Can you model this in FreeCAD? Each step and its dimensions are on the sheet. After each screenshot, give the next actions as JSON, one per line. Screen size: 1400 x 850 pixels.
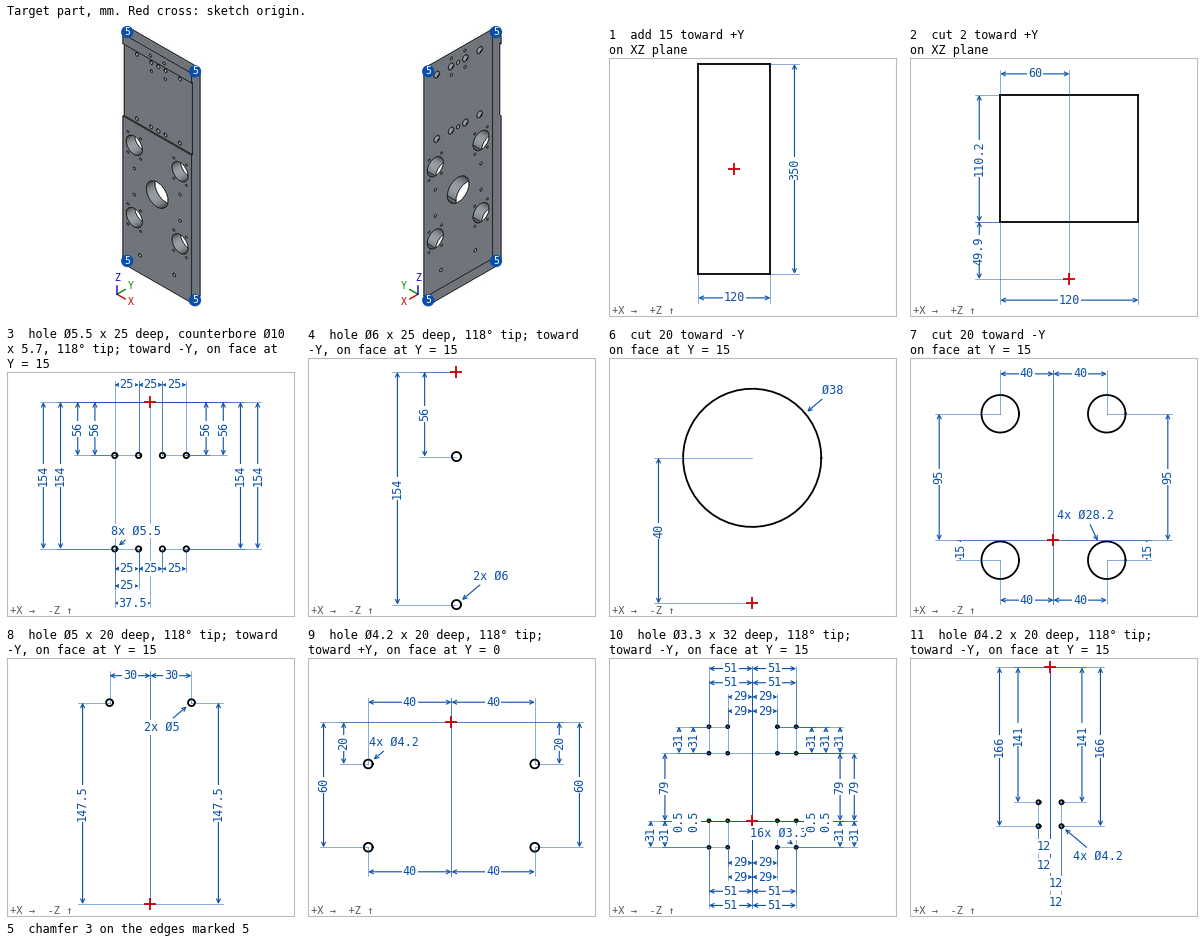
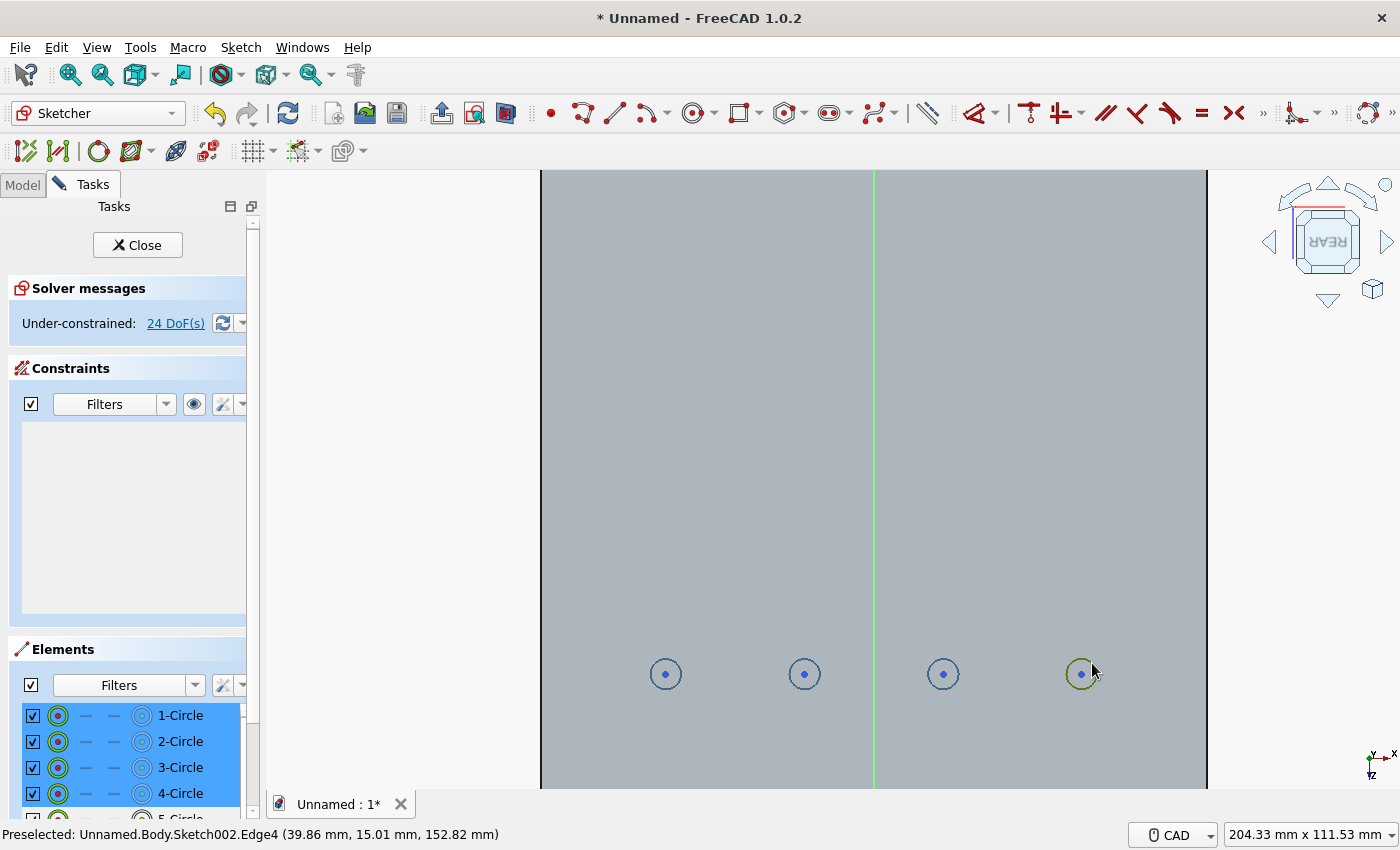
{"action": "scroll", "coordinate": [675, 664], "scroll_direction": "down", "scroll_amount": 4}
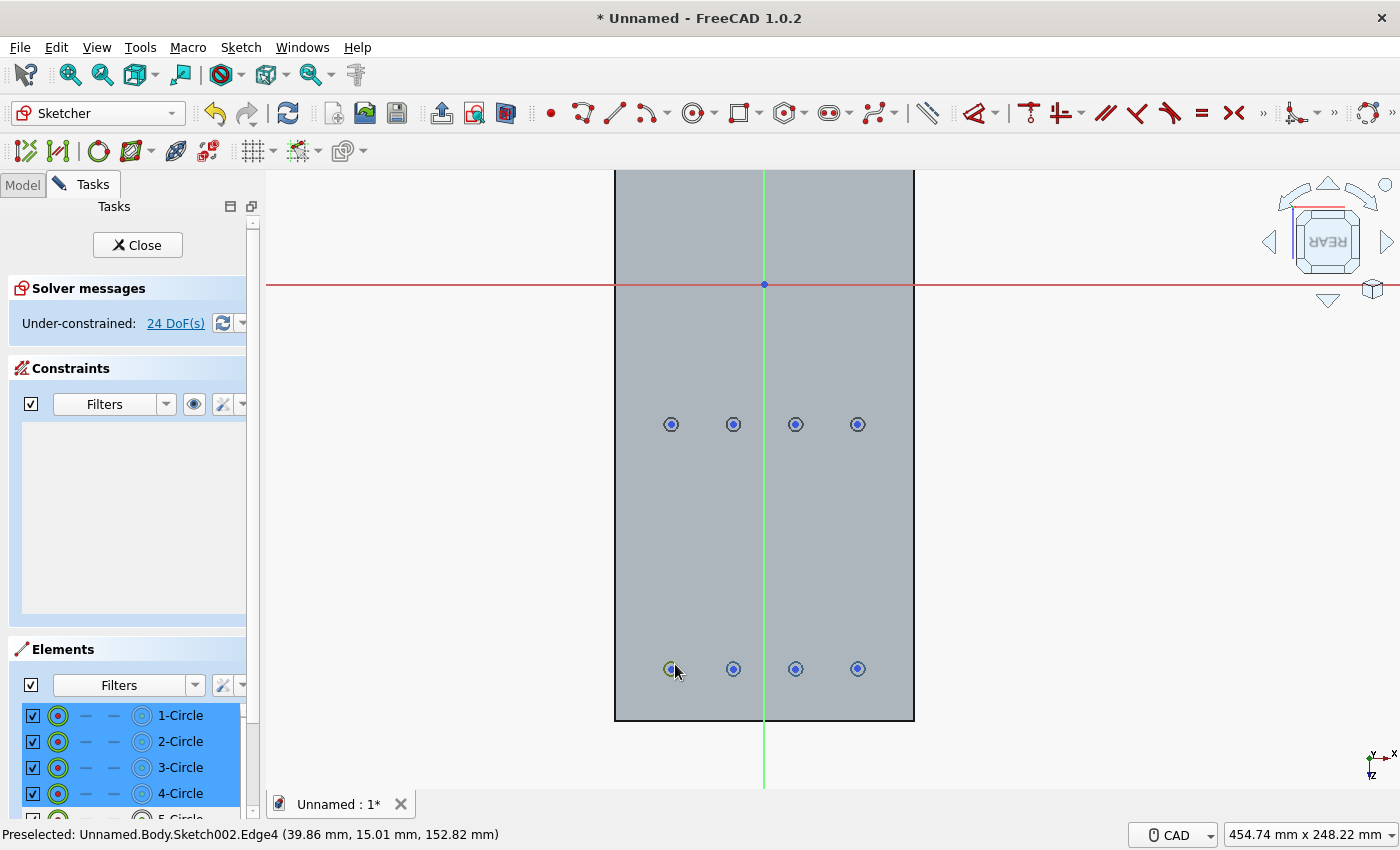
{"action": "scroll", "coordinate": [676, 420], "scroll_direction": "up", "scroll_amount": 4}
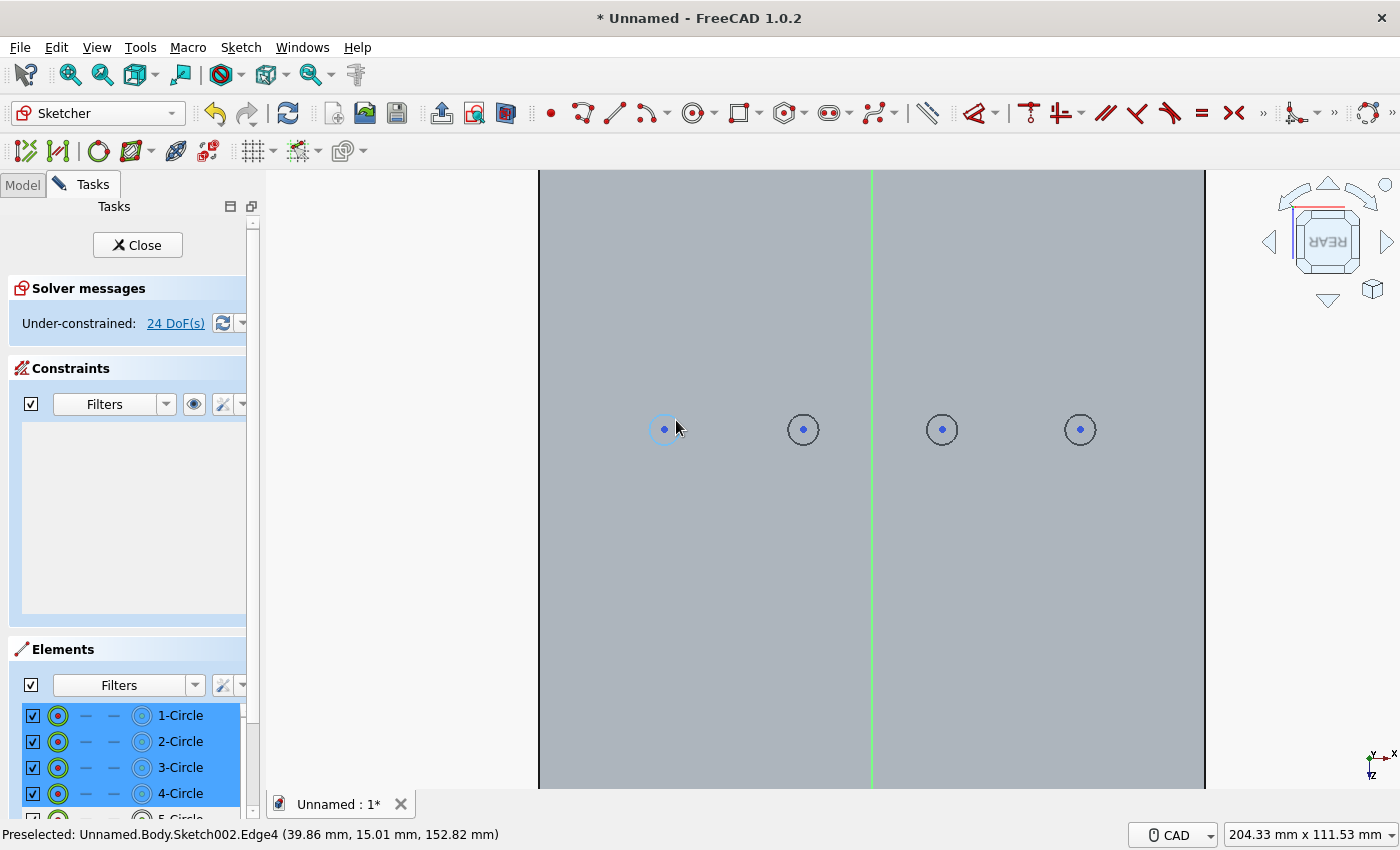
{"action": "left_click", "coordinate": [675, 419]}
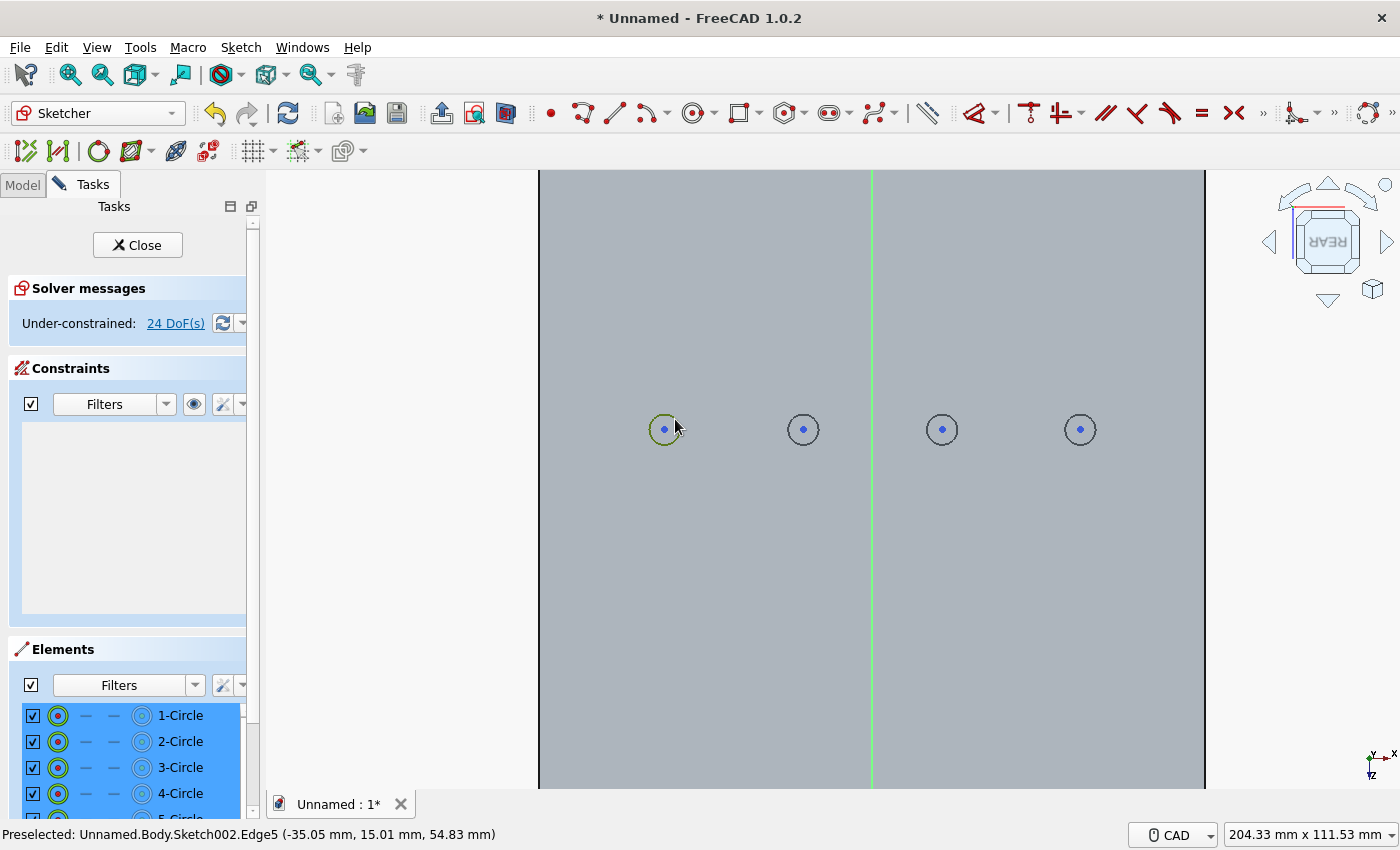
{"action": "left_click", "coordinate": [814, 419]}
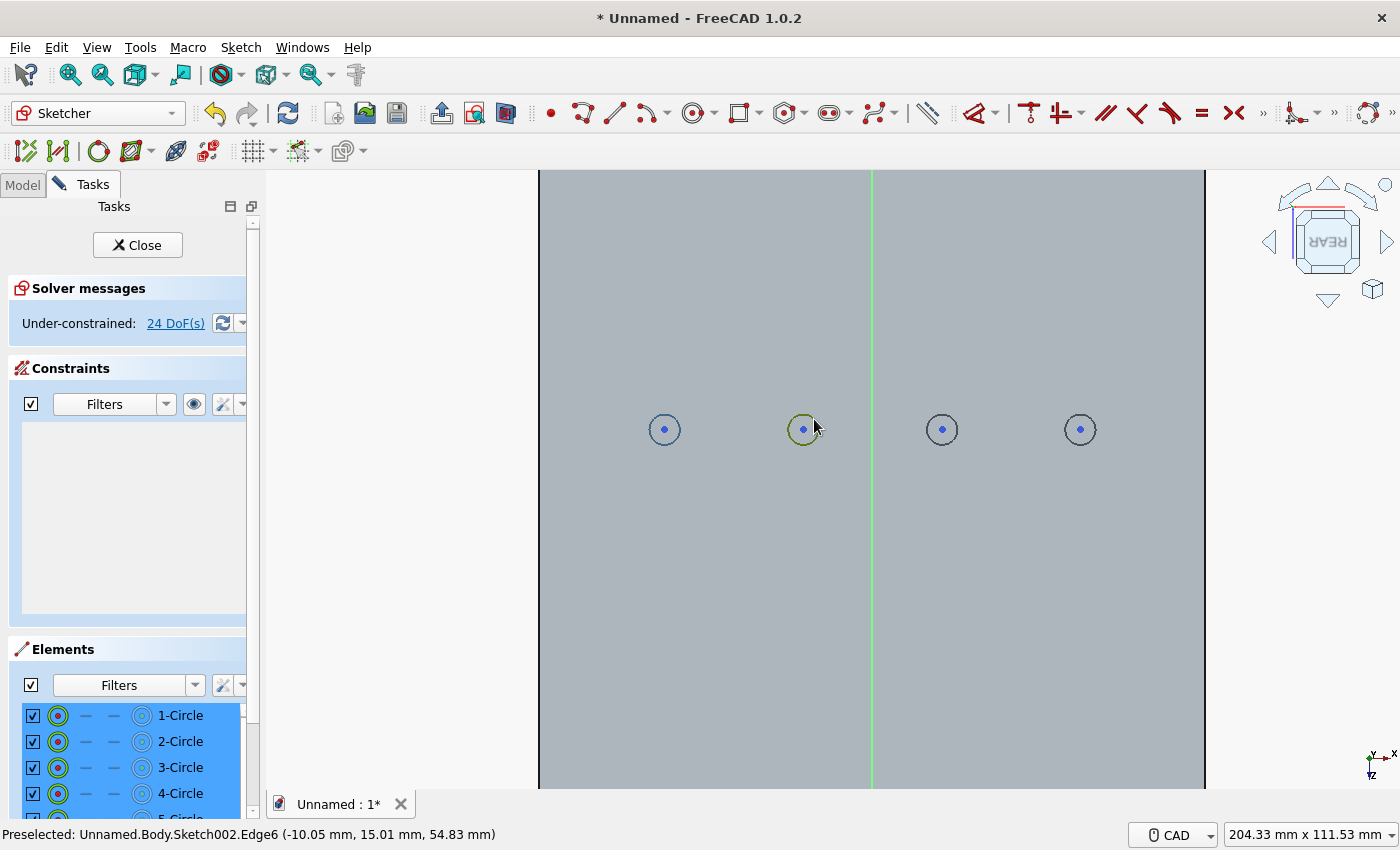
{"action": "left_click", "coordinate": [953, 419]}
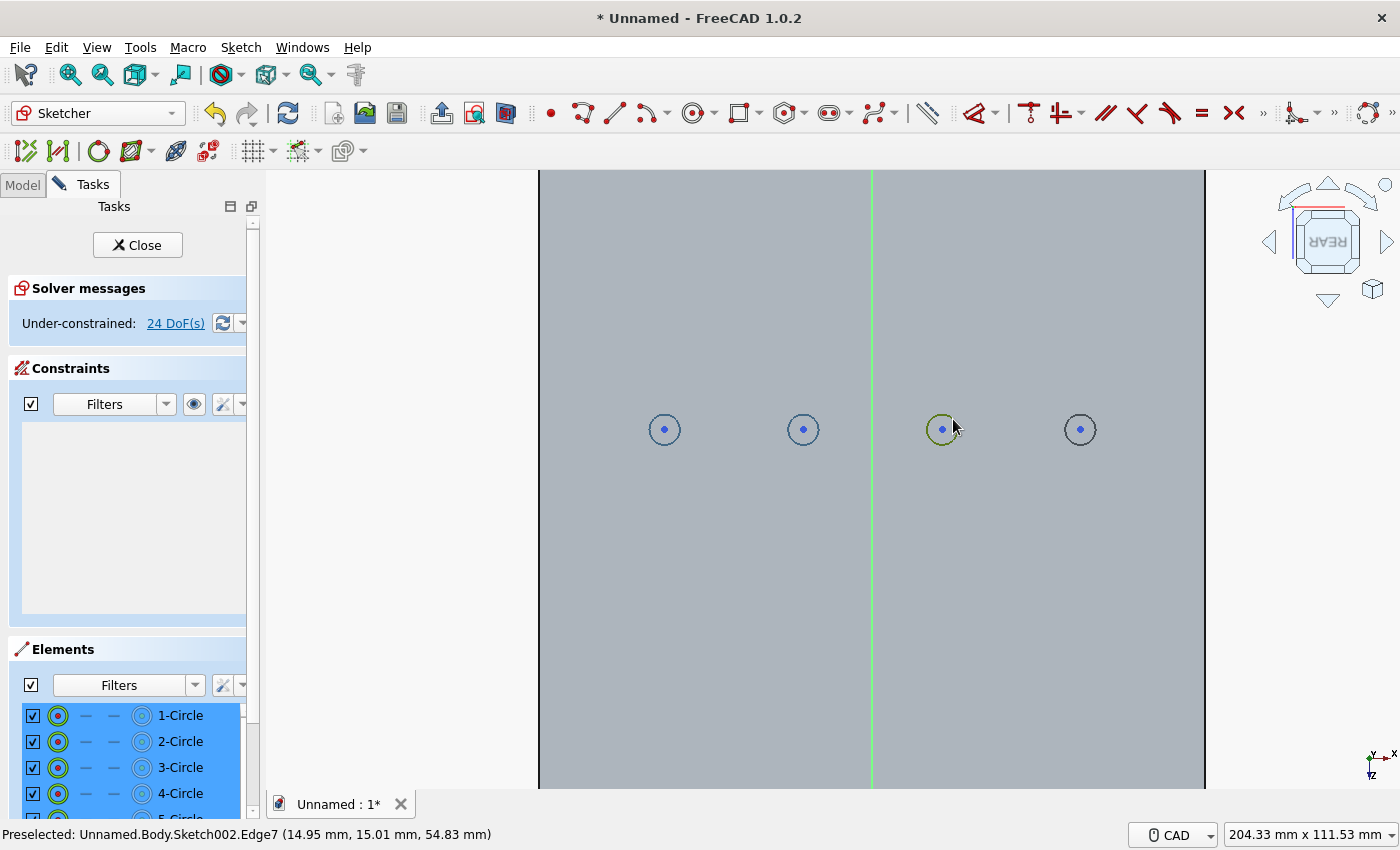
{"action": "left_click", "coordinate": [1091, 419]}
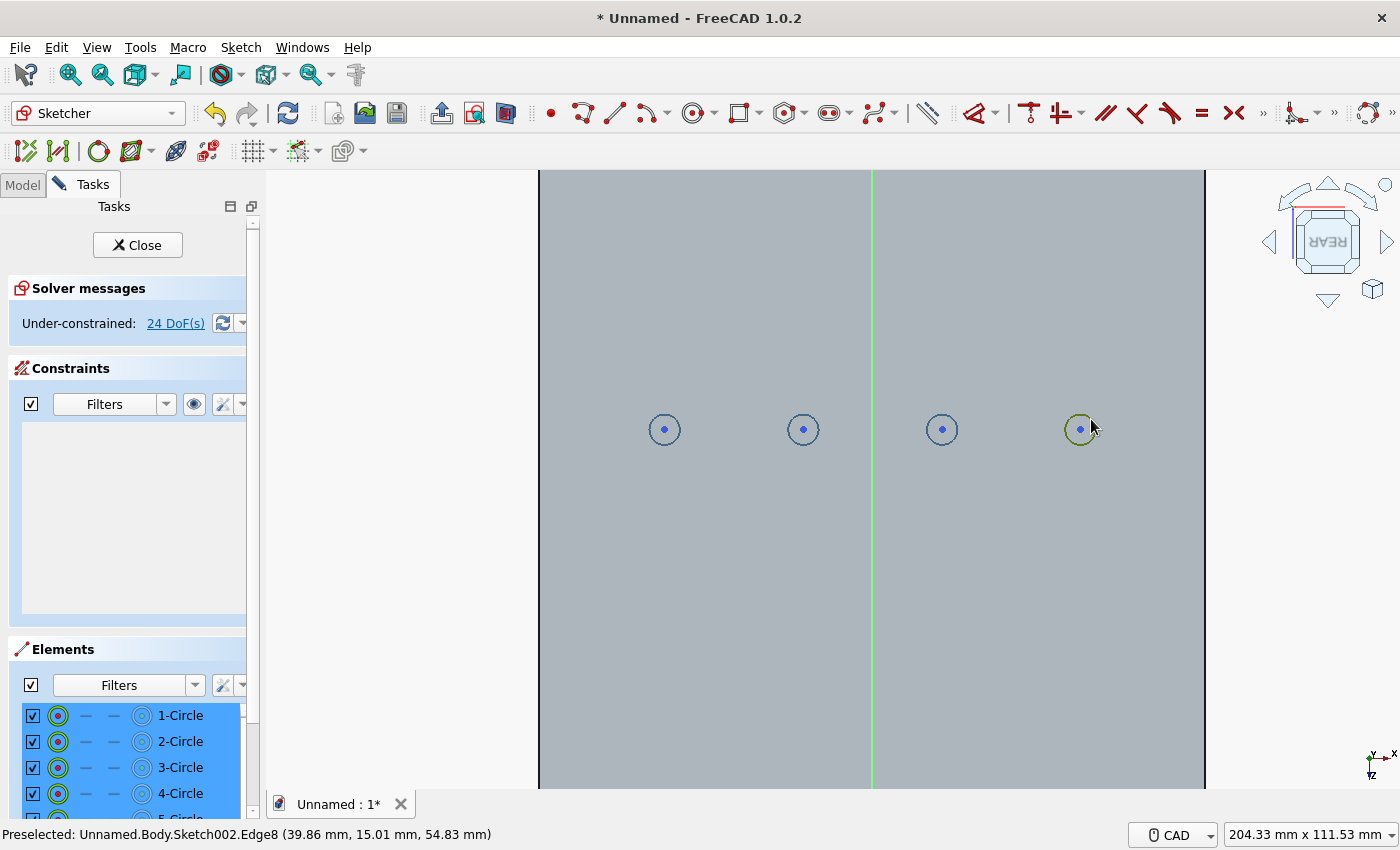
{"action": "left_click", "coordinate": [1202, 114]}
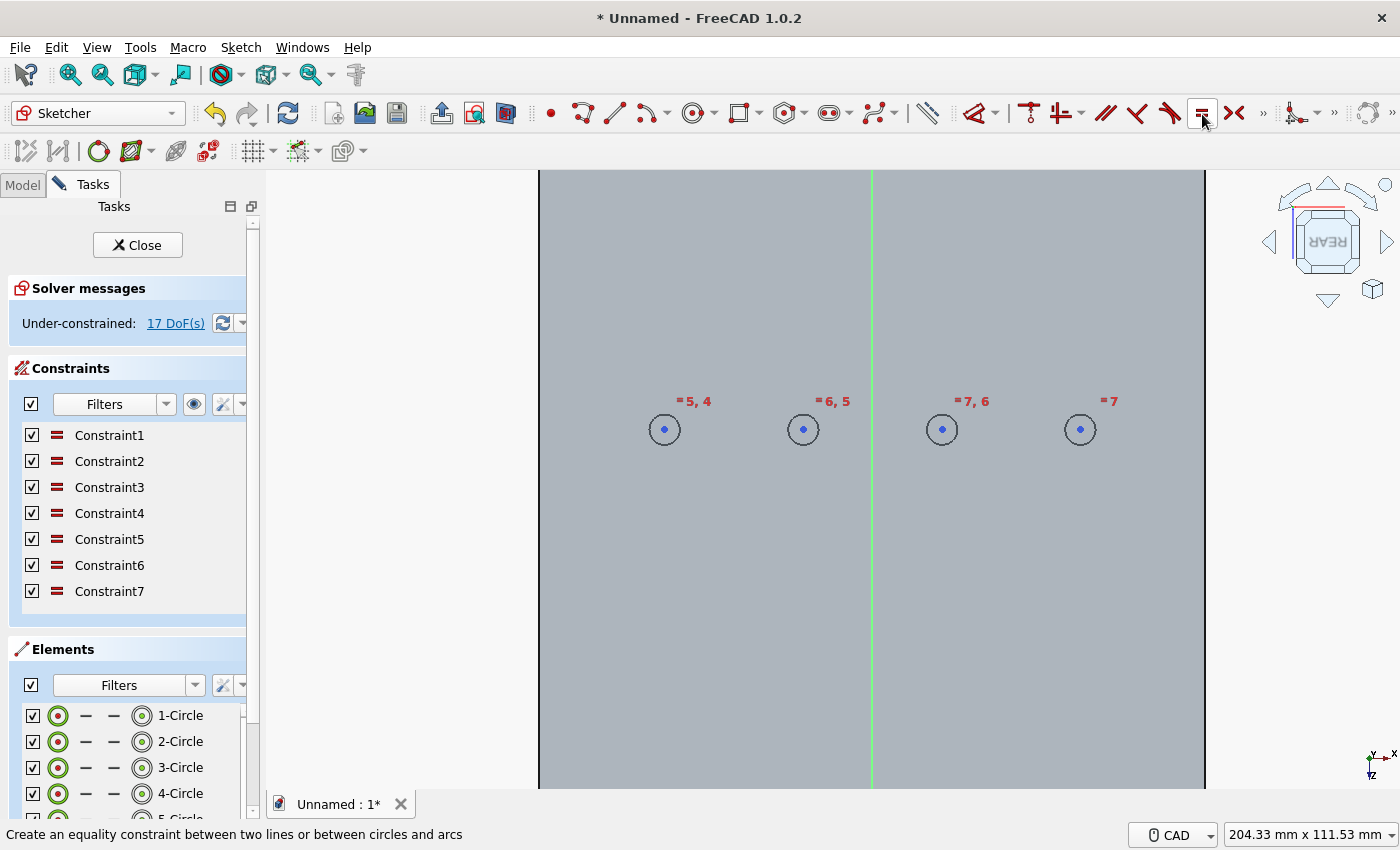
{"action": "key", "text": "d"}